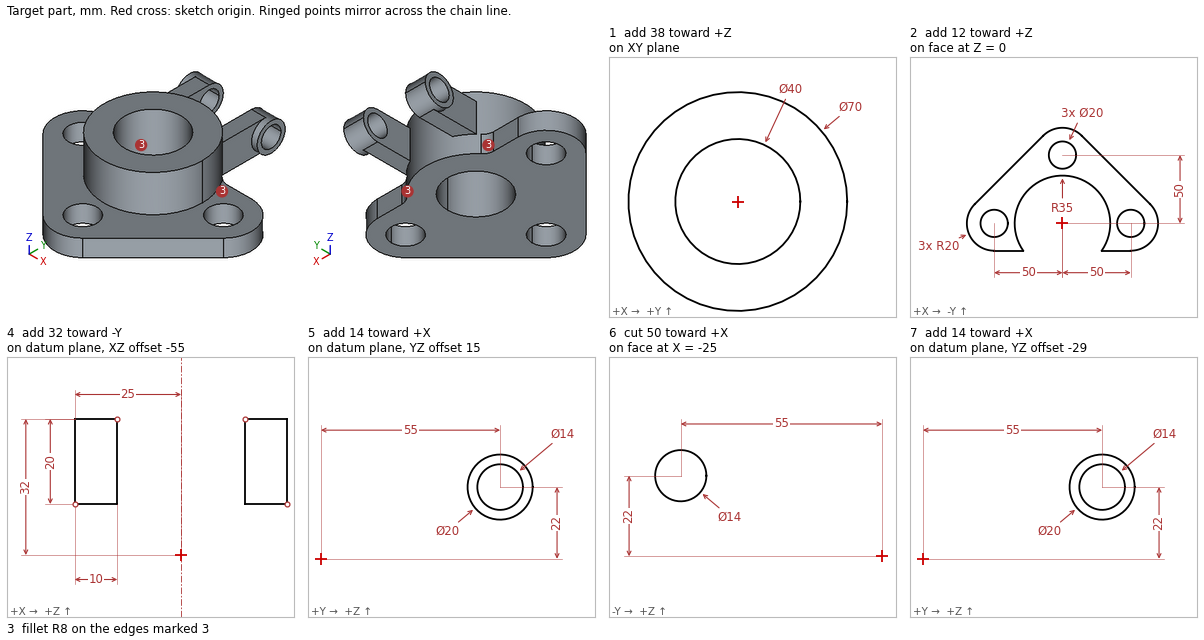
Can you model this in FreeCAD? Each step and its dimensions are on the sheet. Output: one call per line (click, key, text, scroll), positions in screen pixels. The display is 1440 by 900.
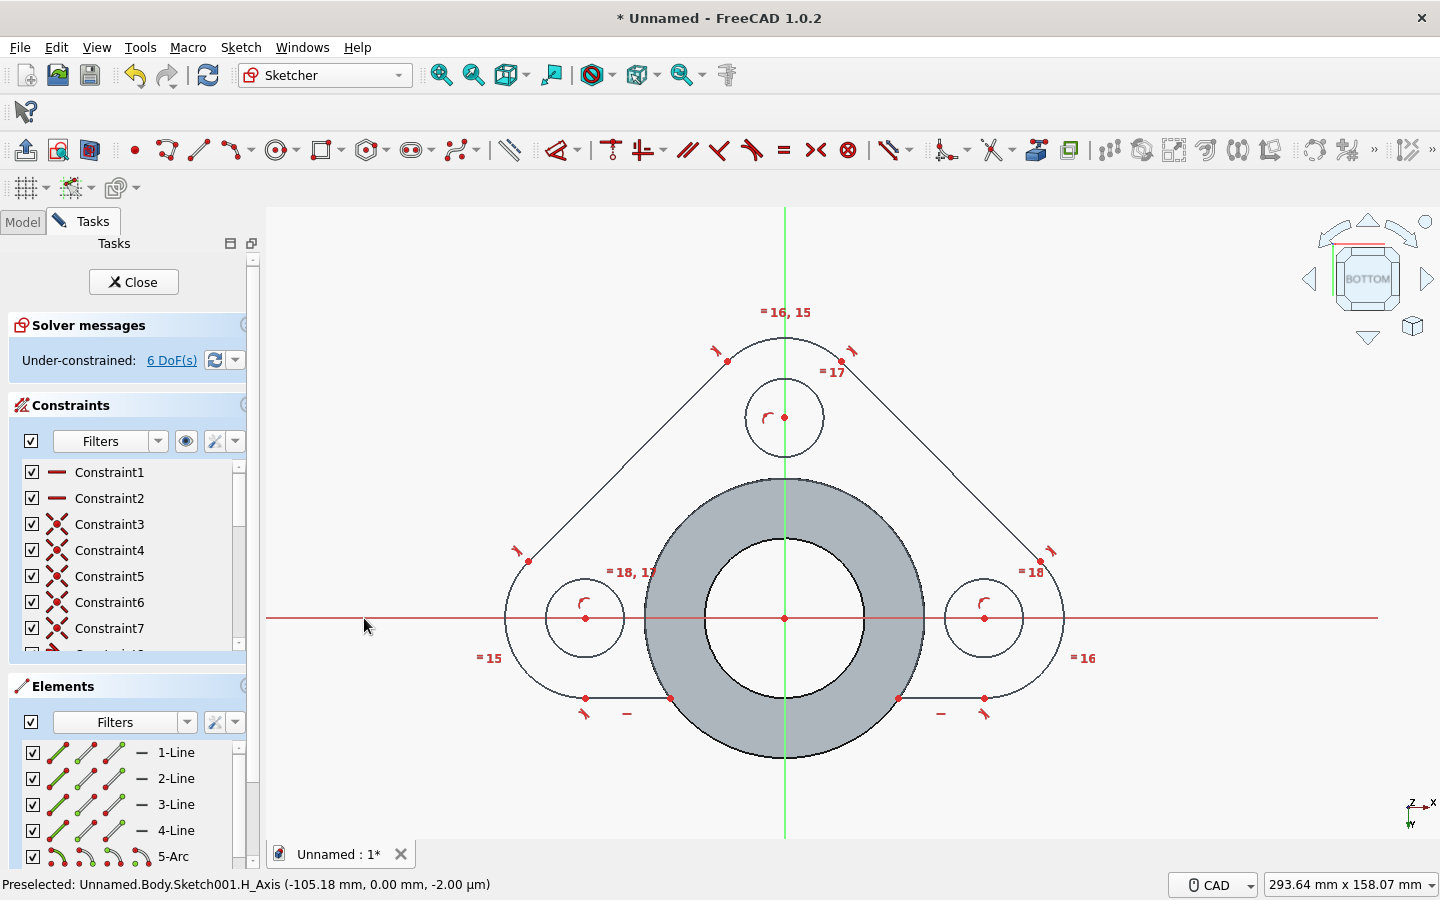
key(d)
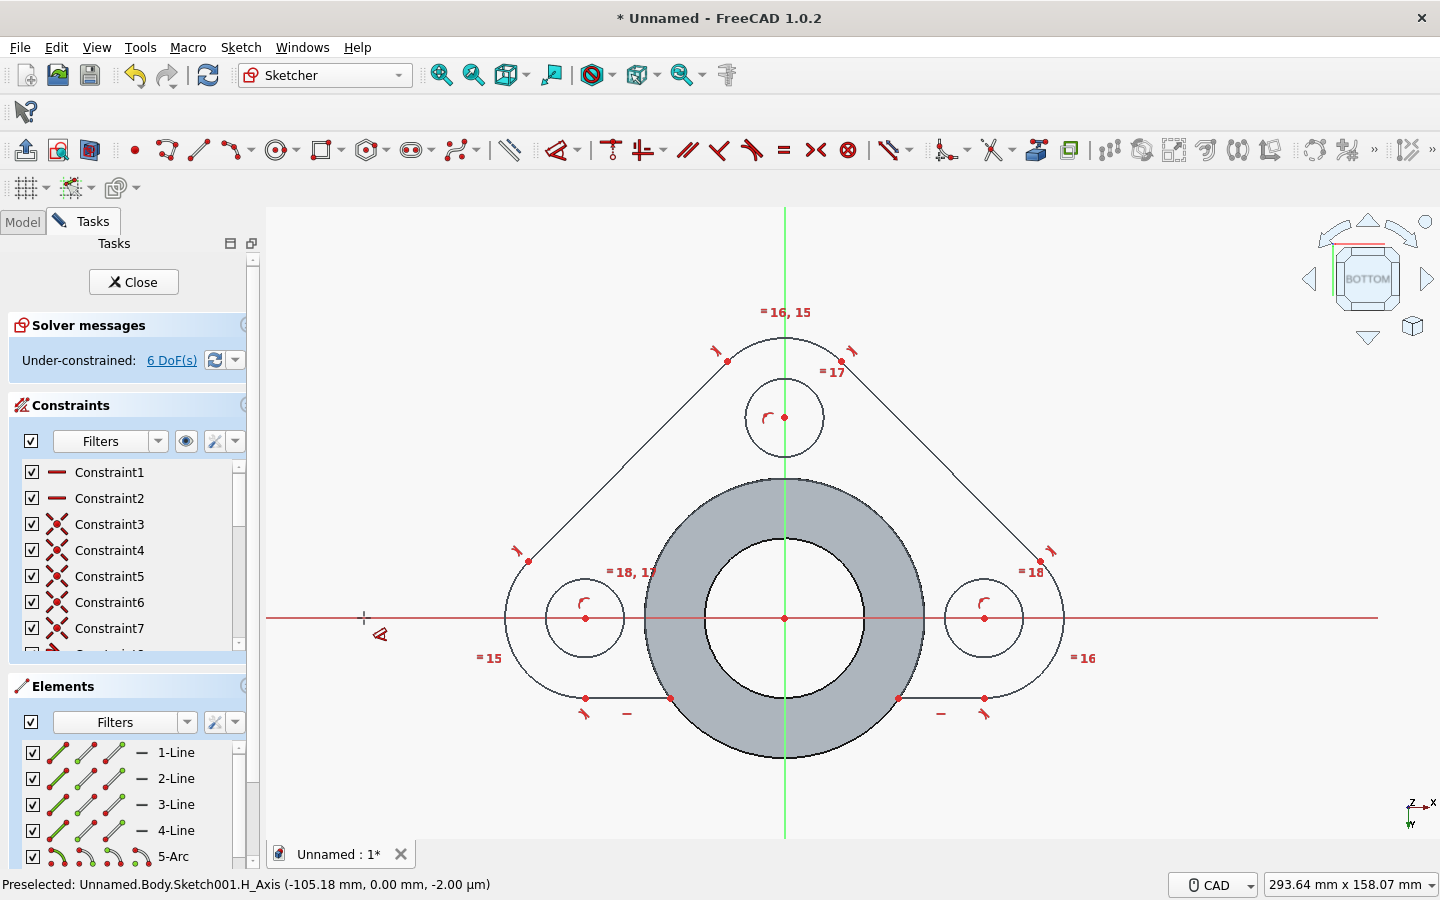
click(891, 529)
click(916, 508)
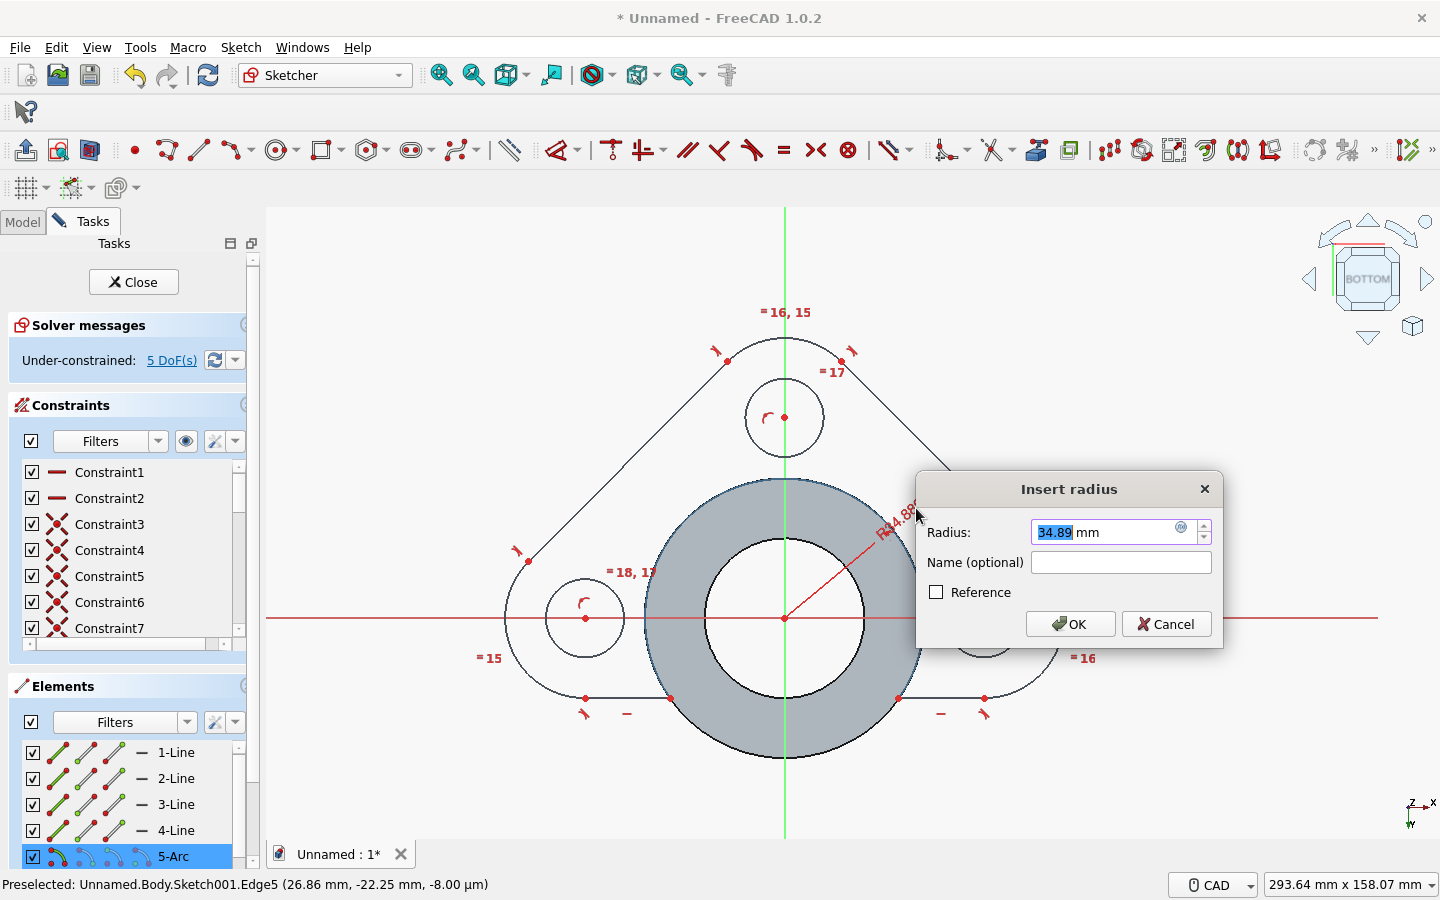
text(35)
key(Return)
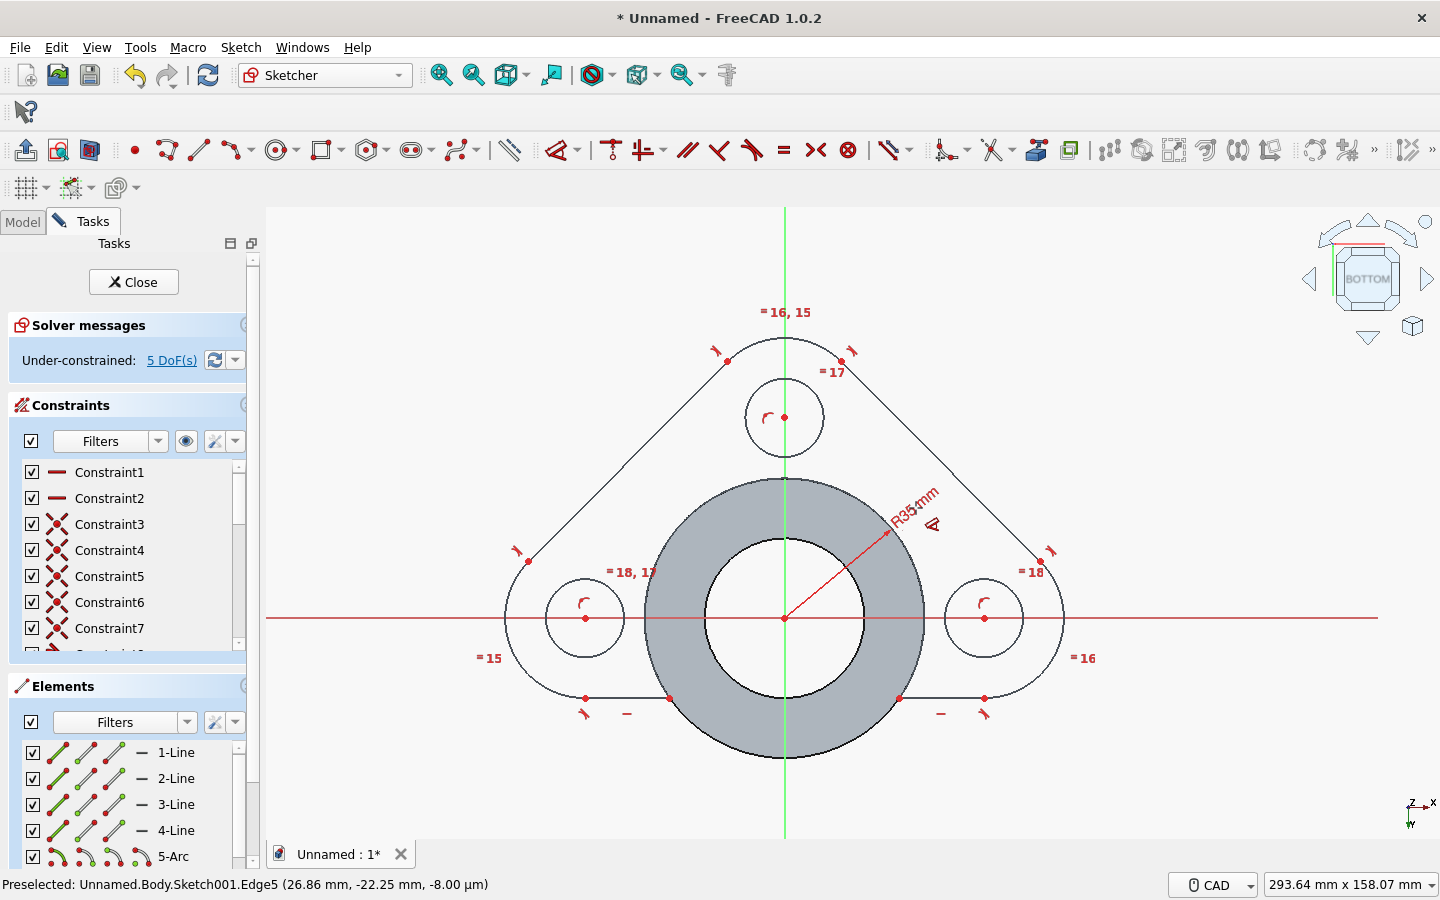
click(533, 679)
click(512, 703)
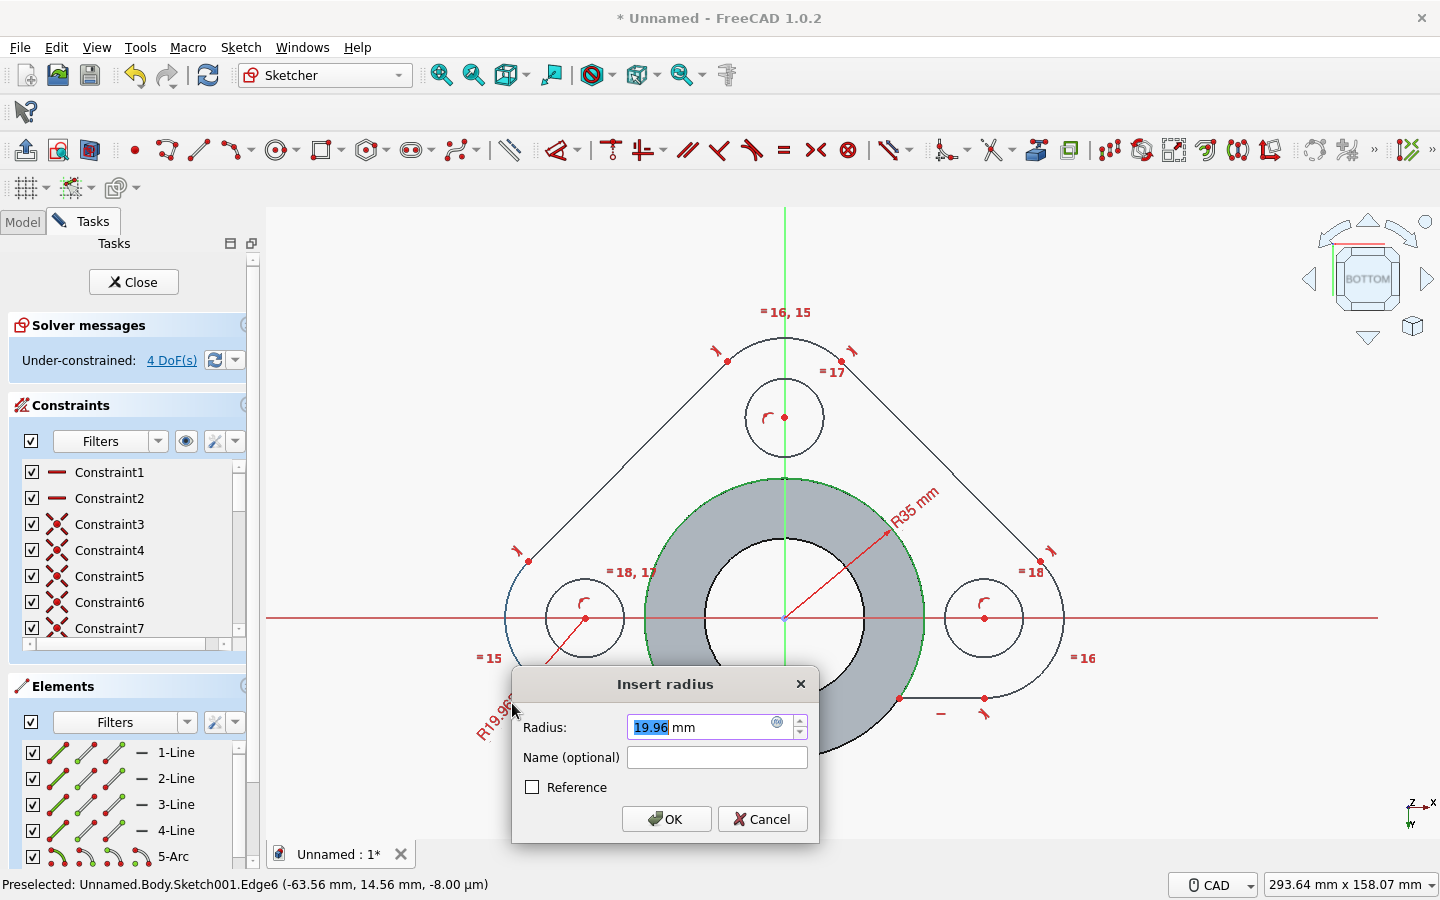
text(20)
key(Return)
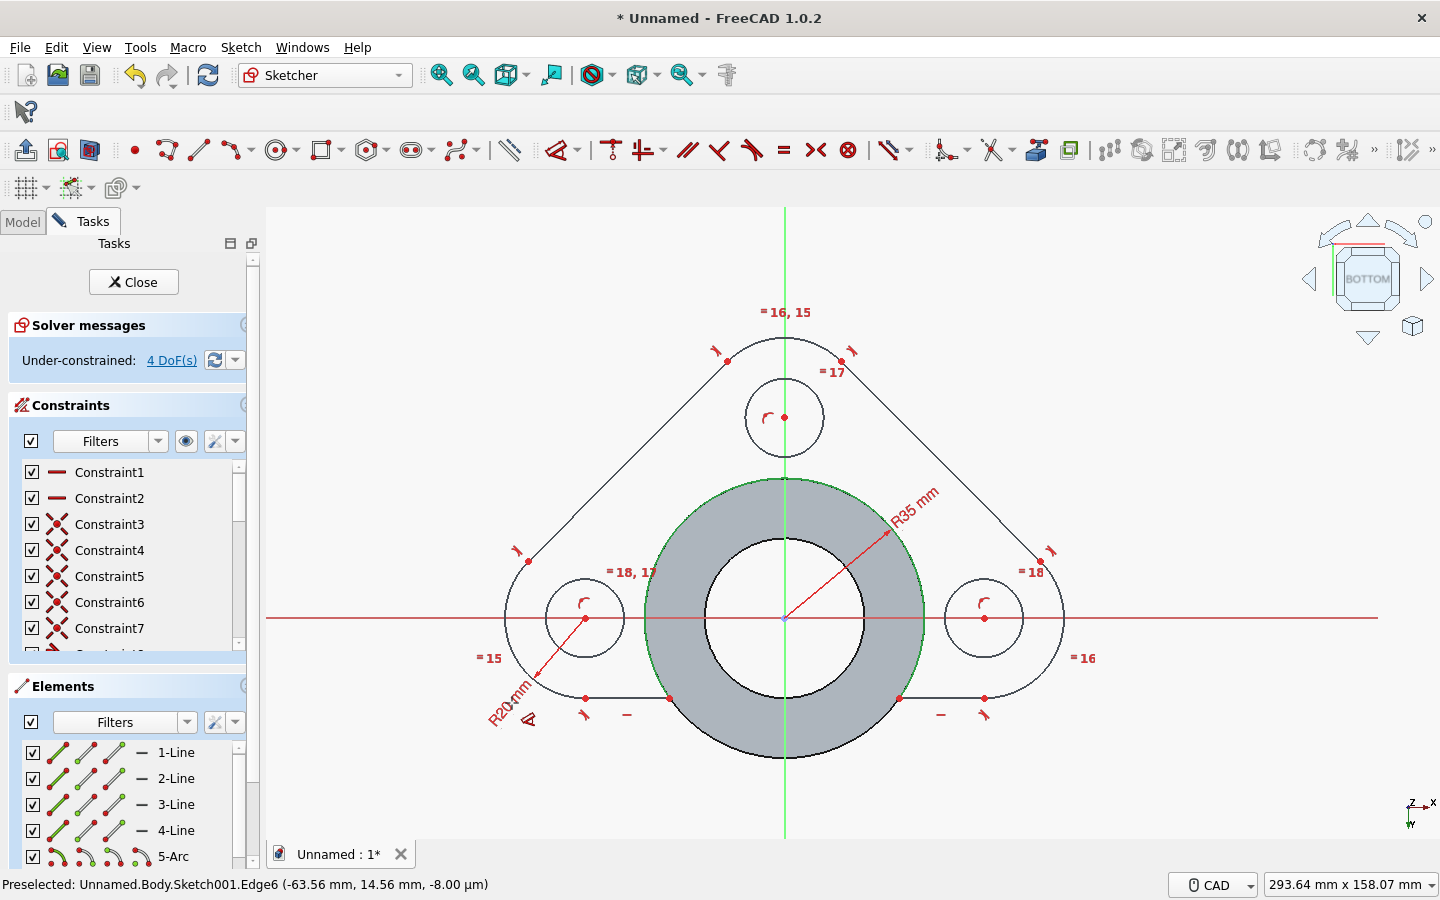
click(812, 390)
click(853, 397)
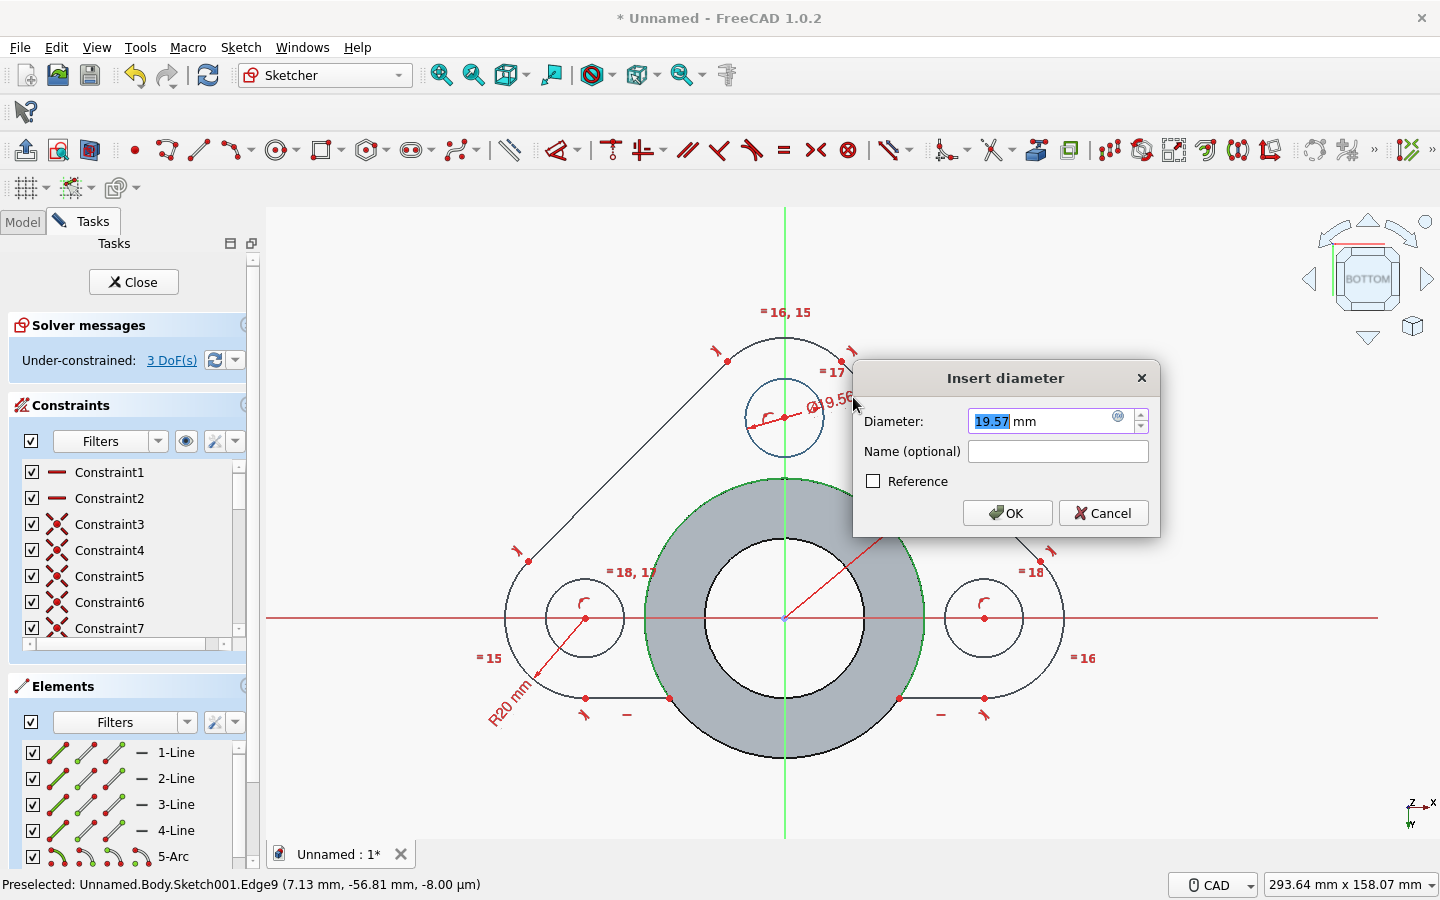
text(20)
key(Return)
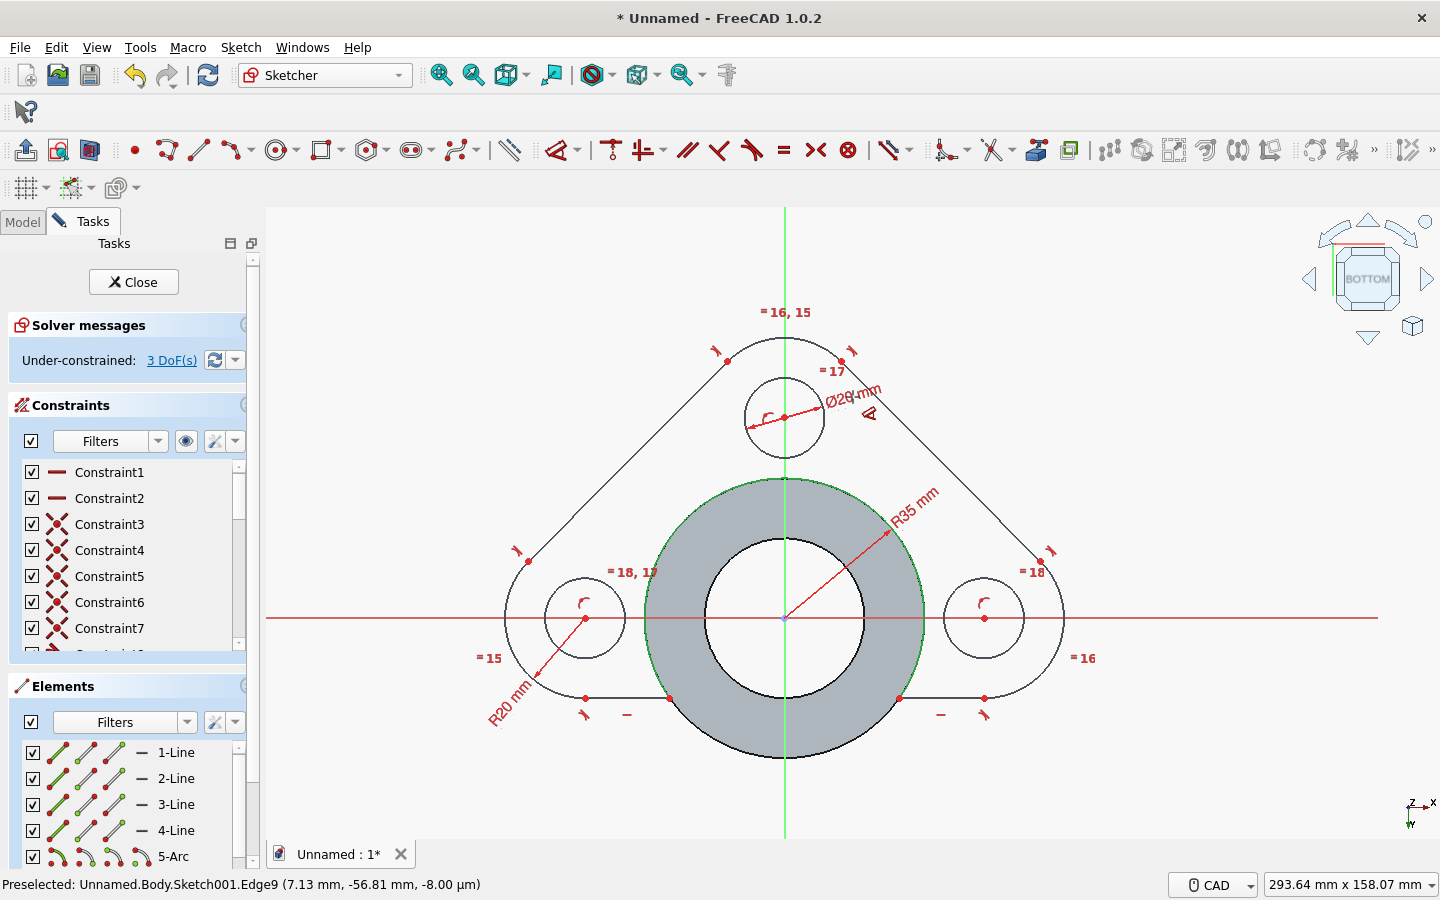
click(785, 418)
click(819, 518)